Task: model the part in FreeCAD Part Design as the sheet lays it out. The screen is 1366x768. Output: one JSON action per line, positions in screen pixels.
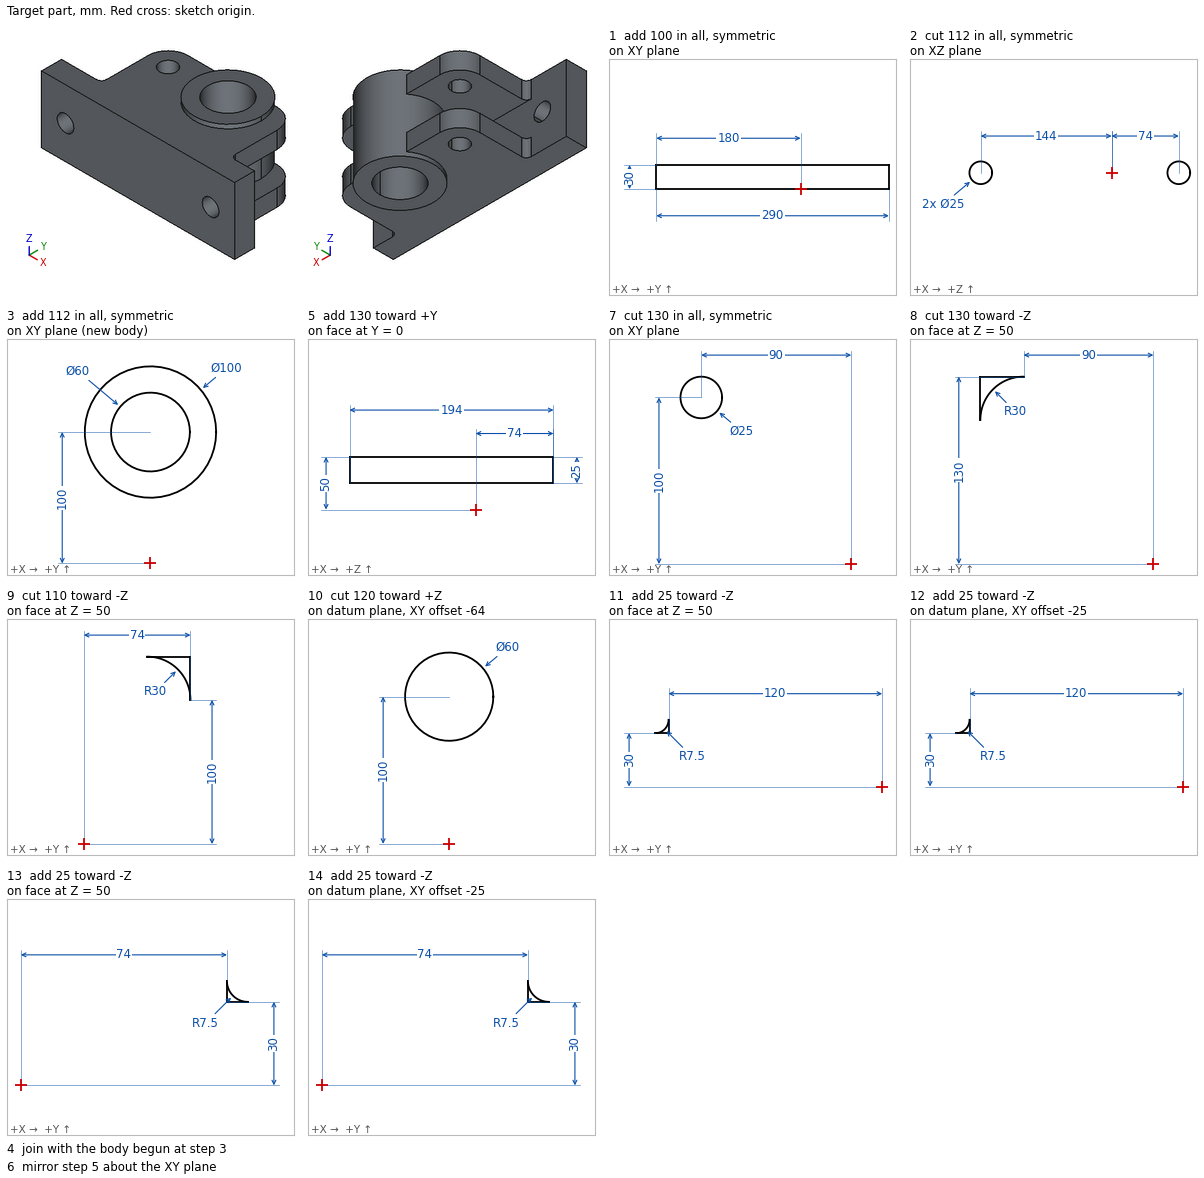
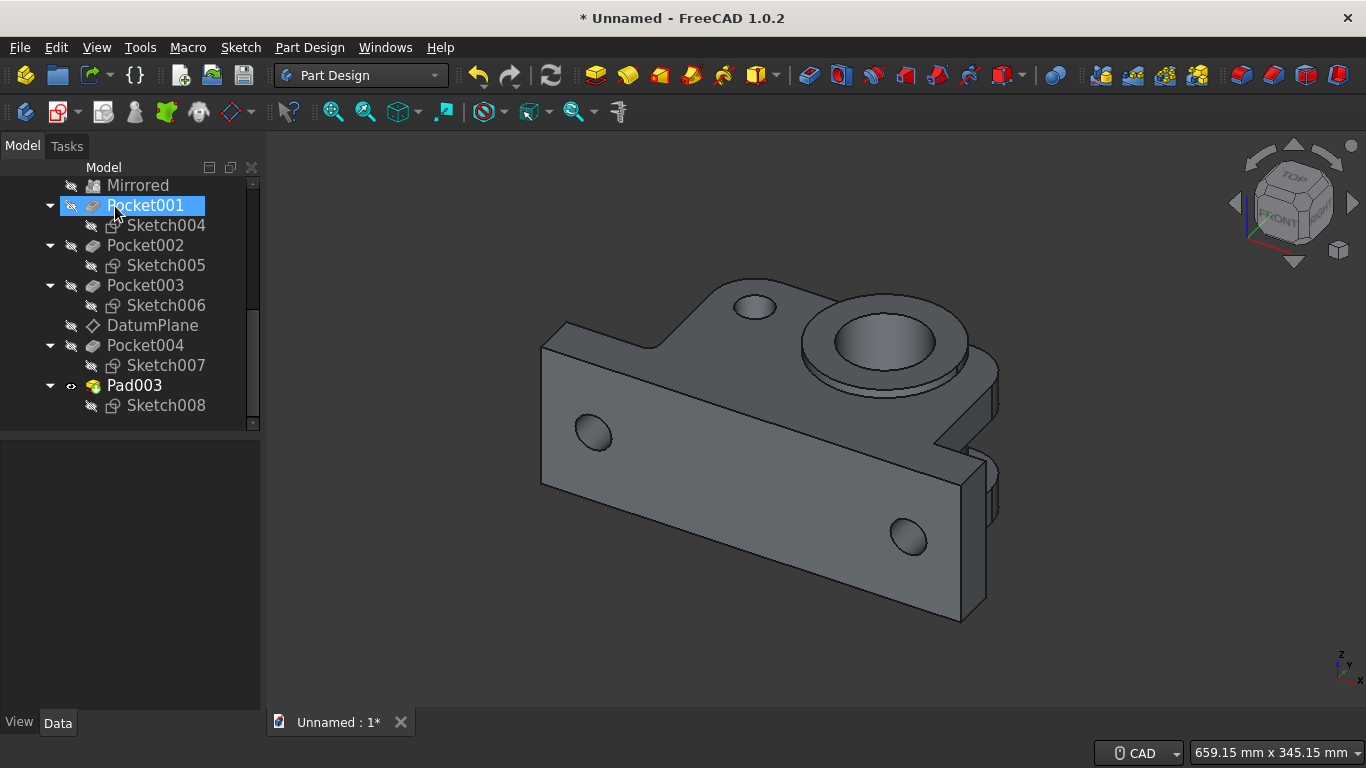
{"action": "scroll", "coordinate": [140, 301], "scroll_direction": "down", "scroll_amount": 3}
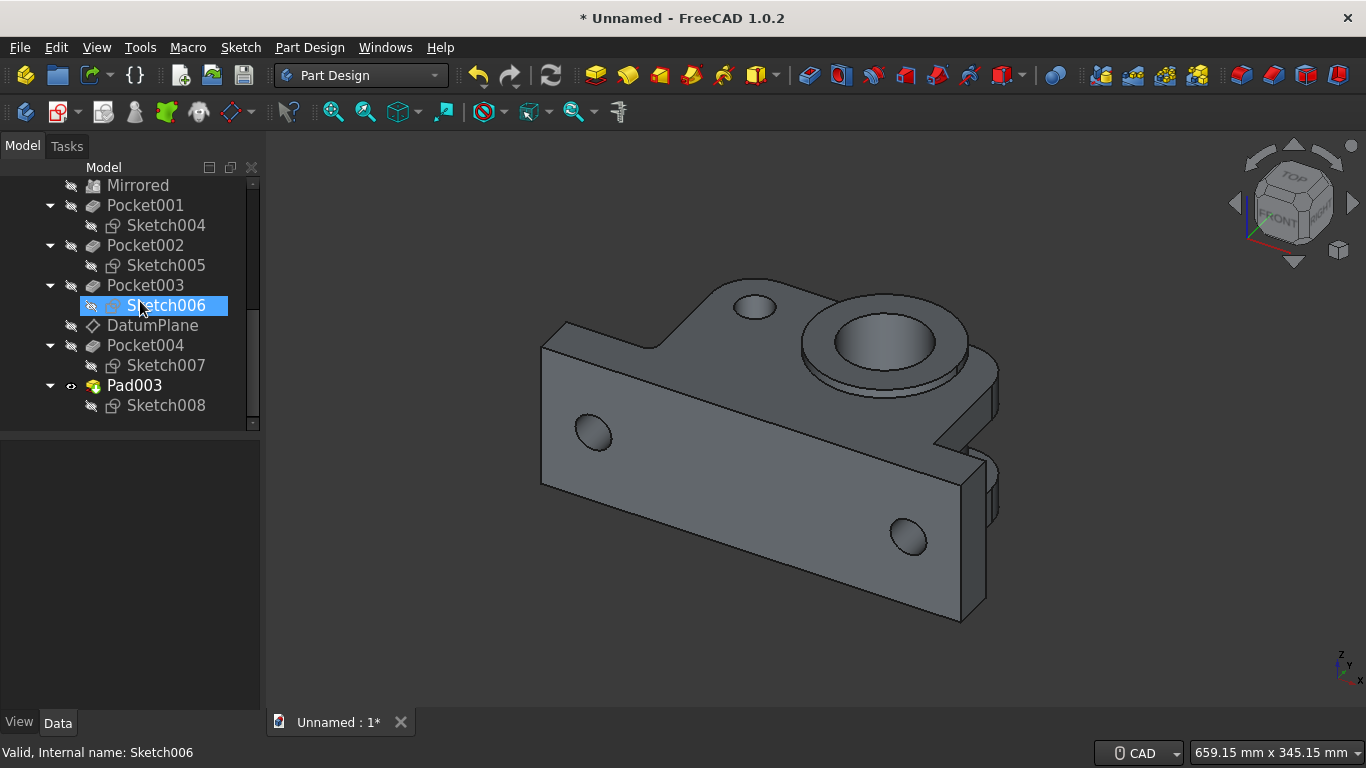
{"action": "scroll", "coordinate": [140, 301], "scroll_direction": "up", "scroll_amount": 15}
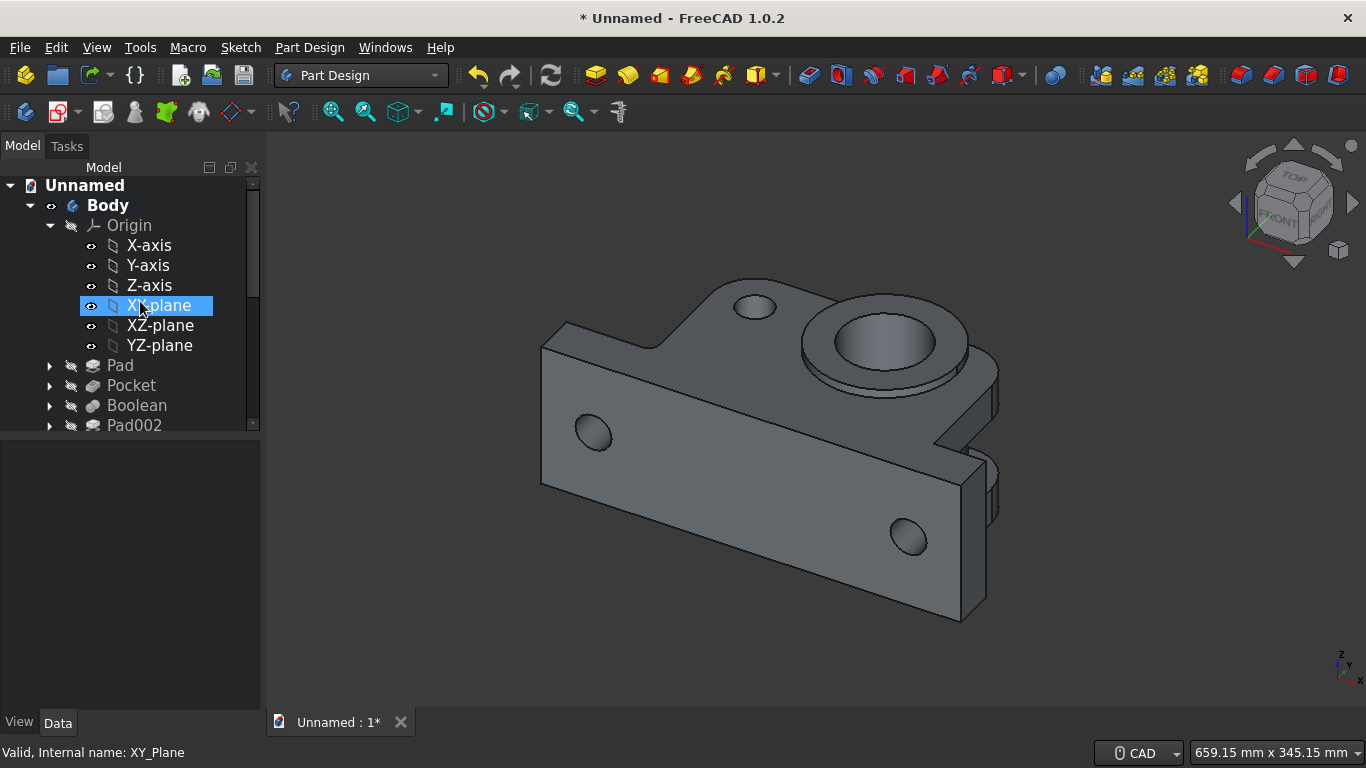
{"action": "left_click", "coordinate": [136, 306]}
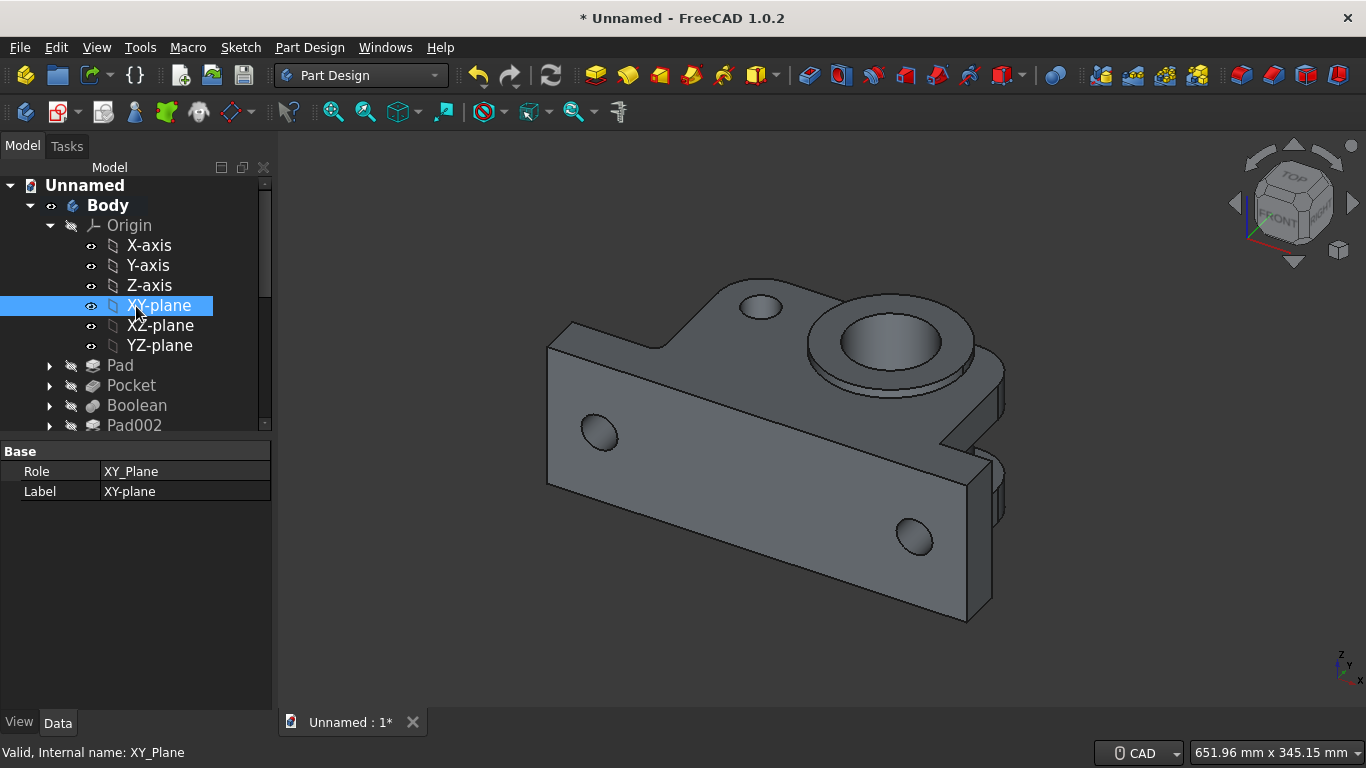
{"action": "left_click", "coordinate": [232, 112]}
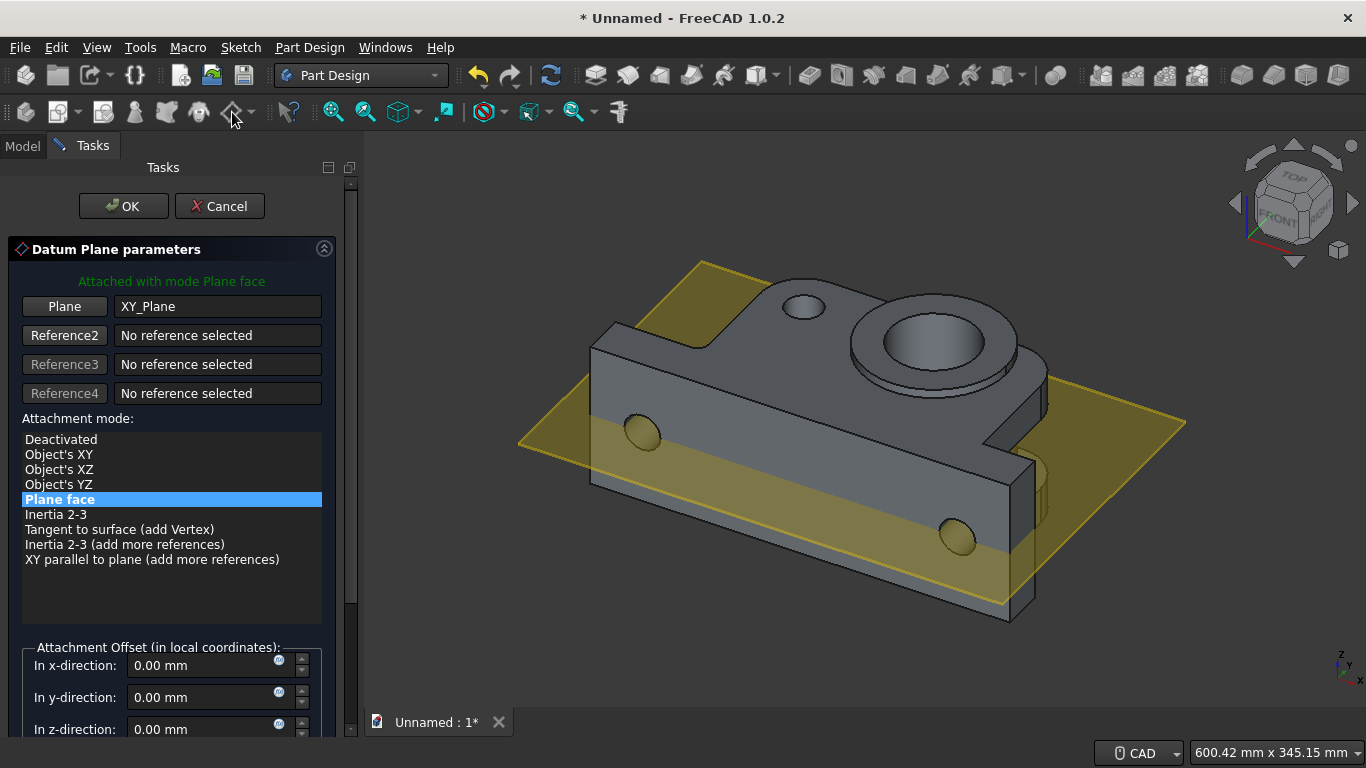
{"action": "scroll", "coordinate": [351, 456], "scroll_direction": "down", "scroll_amount": 2}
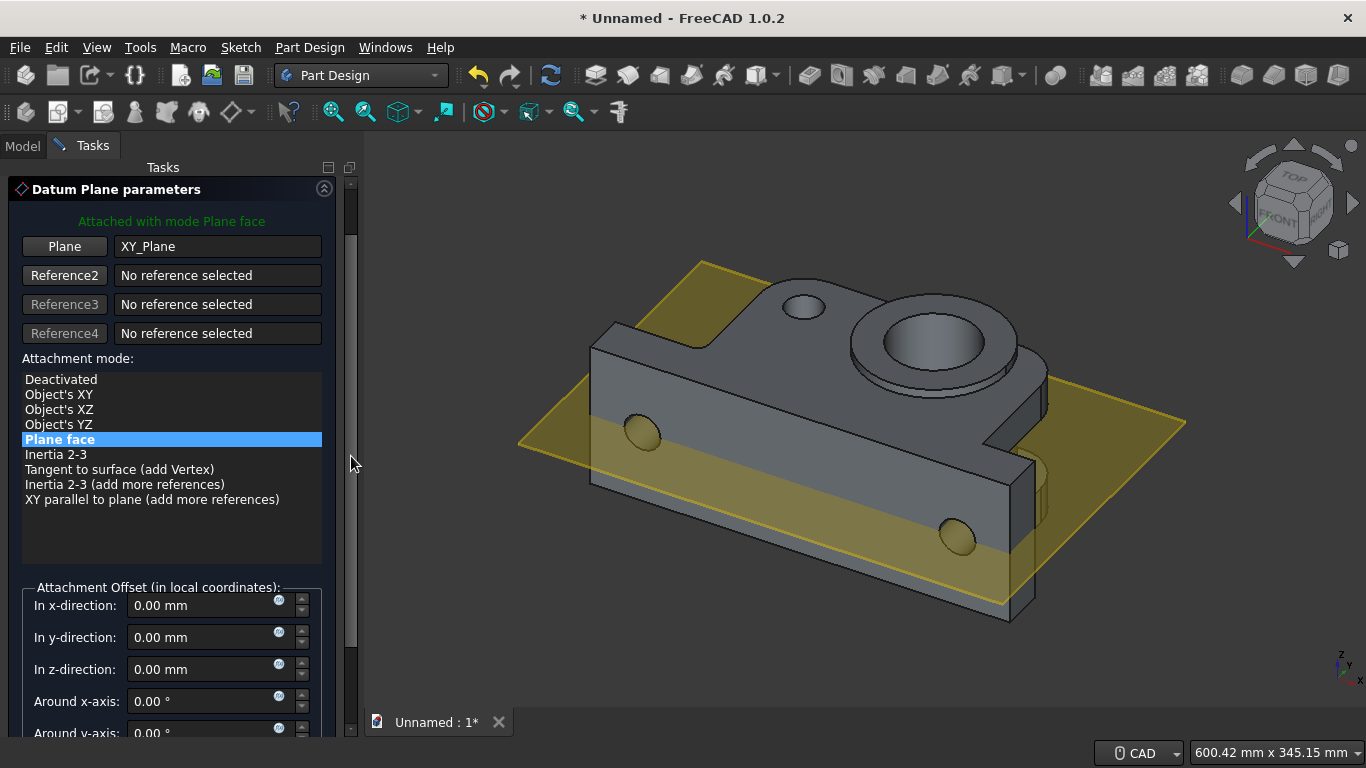
{"action": "triple_click", "coordinate": [210, 609]}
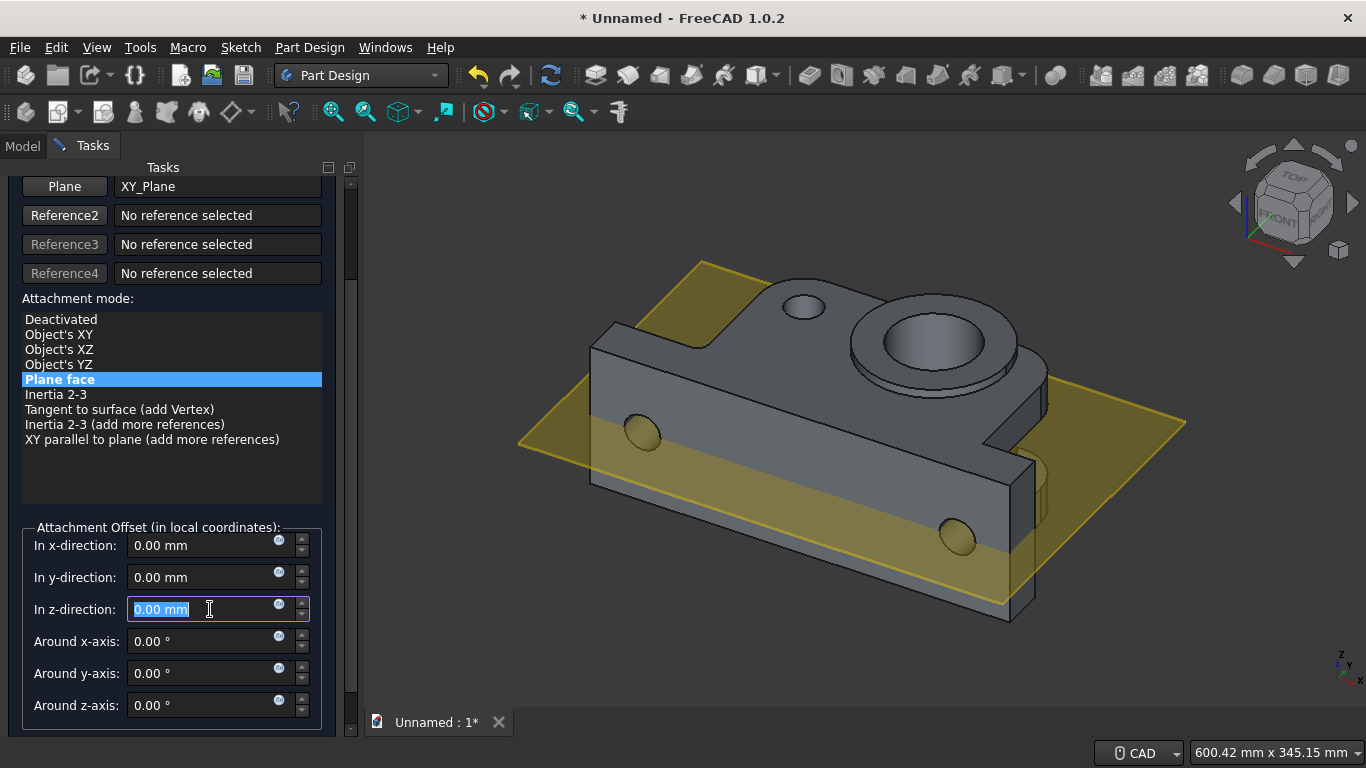
{"action": "type", "text": "-25"}
{"action": "key", "text": "Tab"}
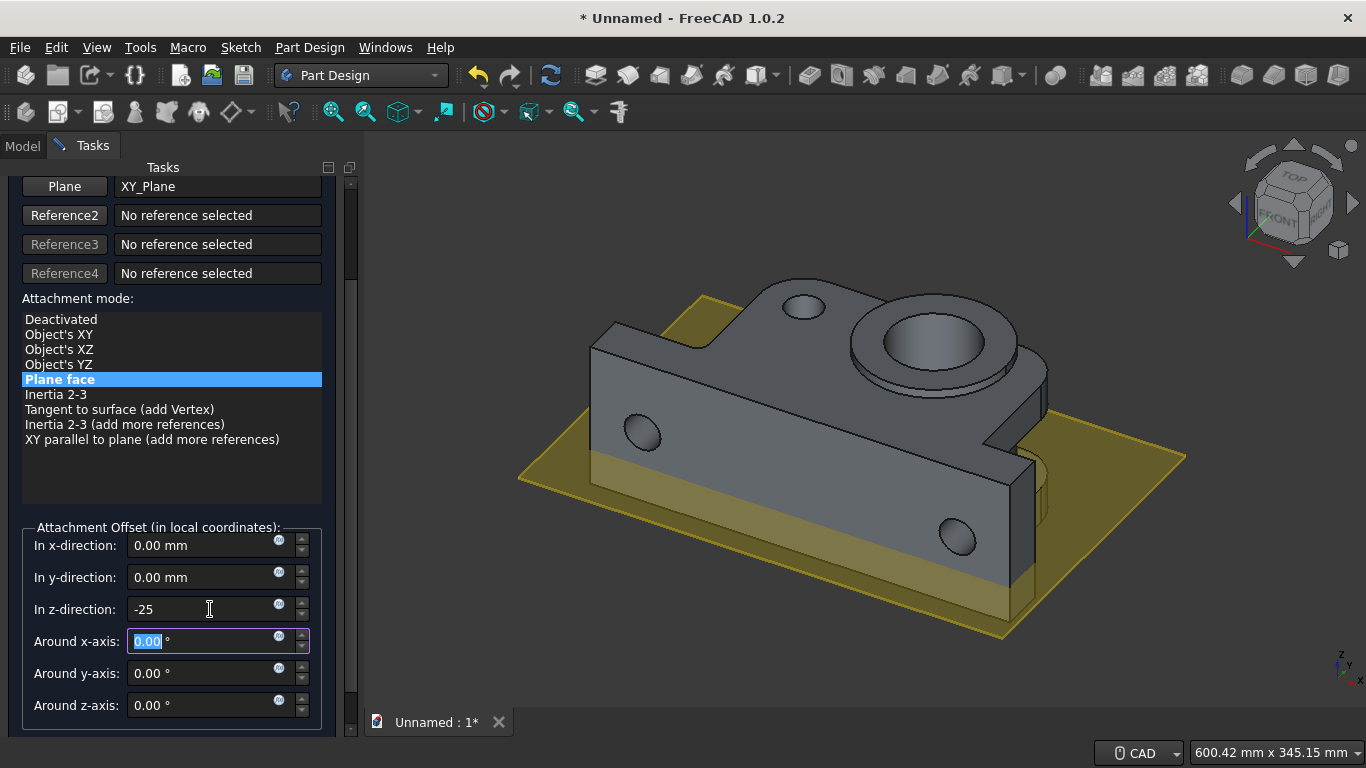
{"action": "scroll", "coordinate": [351, 456], "scroll_direction": "up", "scroll_amount": 3}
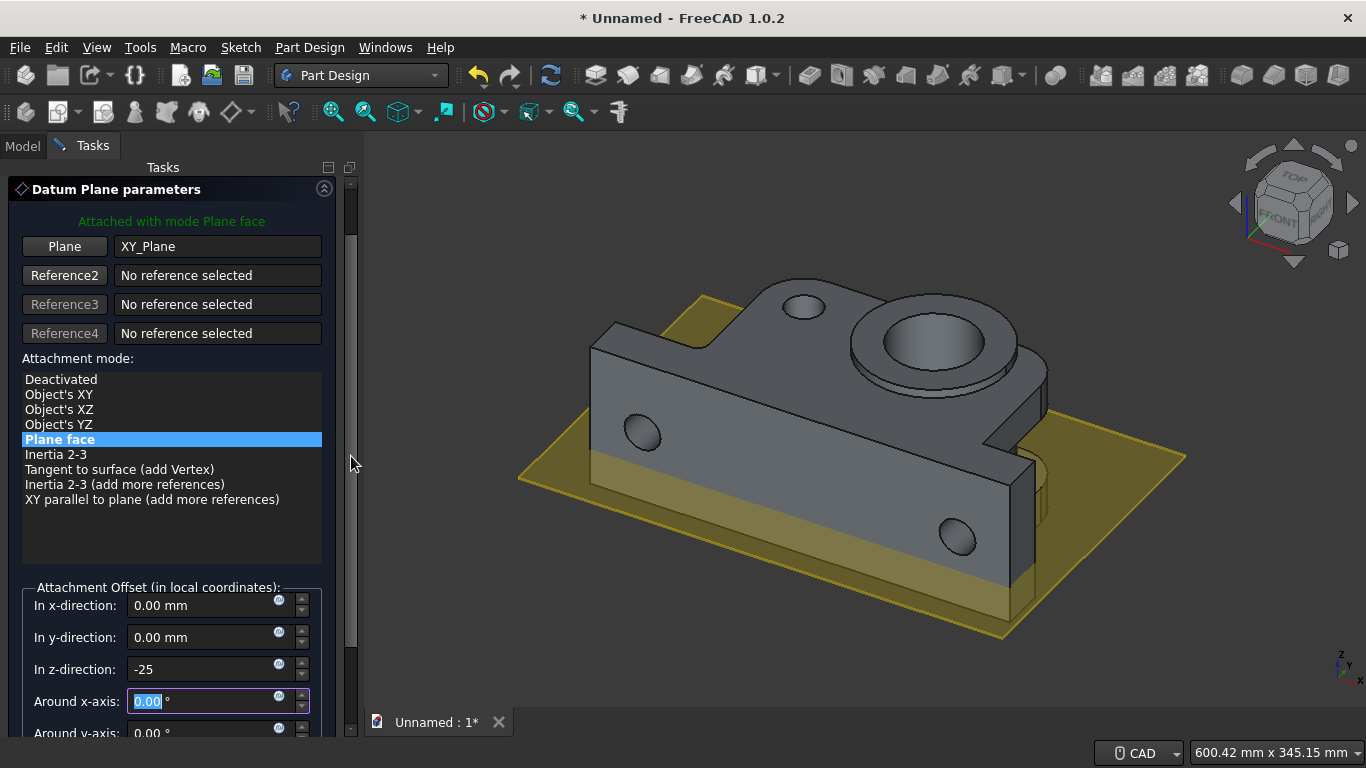
{"action": "left_click", "coordinate": [124, 206]}